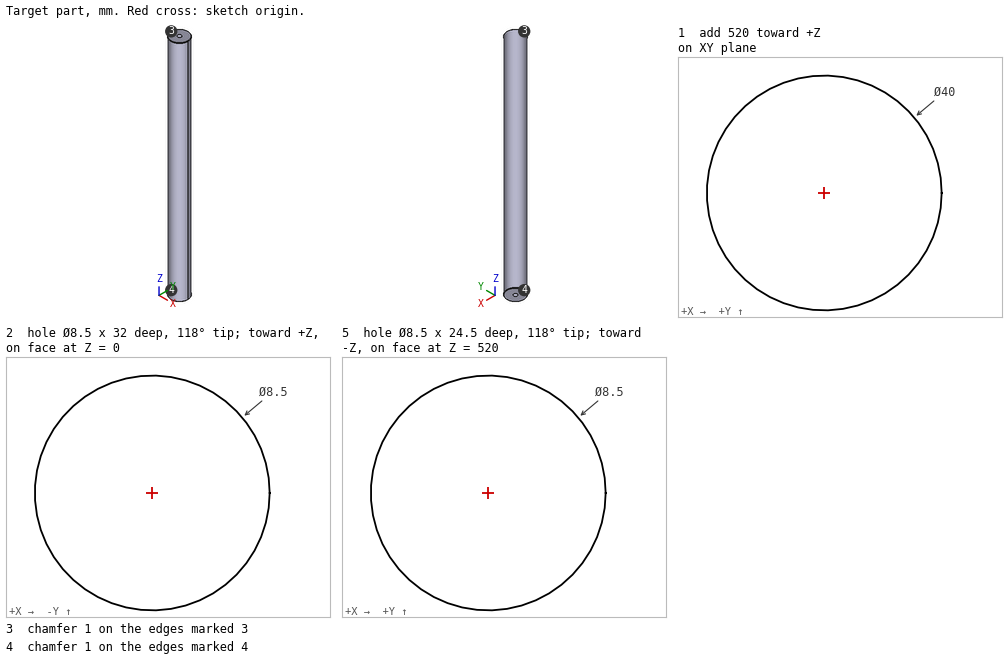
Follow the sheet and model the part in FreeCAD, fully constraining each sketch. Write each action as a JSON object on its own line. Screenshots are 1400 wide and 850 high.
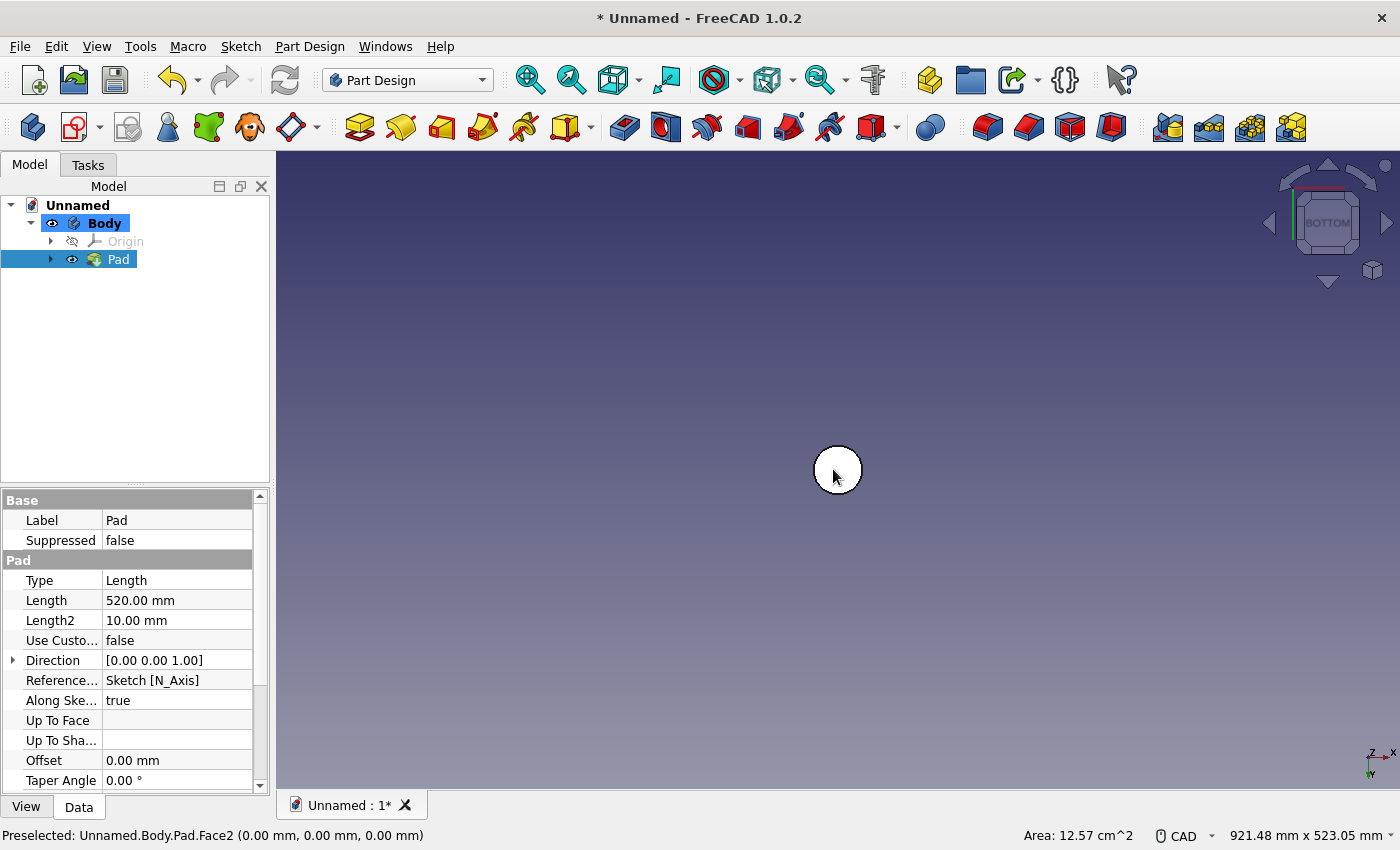
{"action": "left_click", "coordinate": [74, 128]}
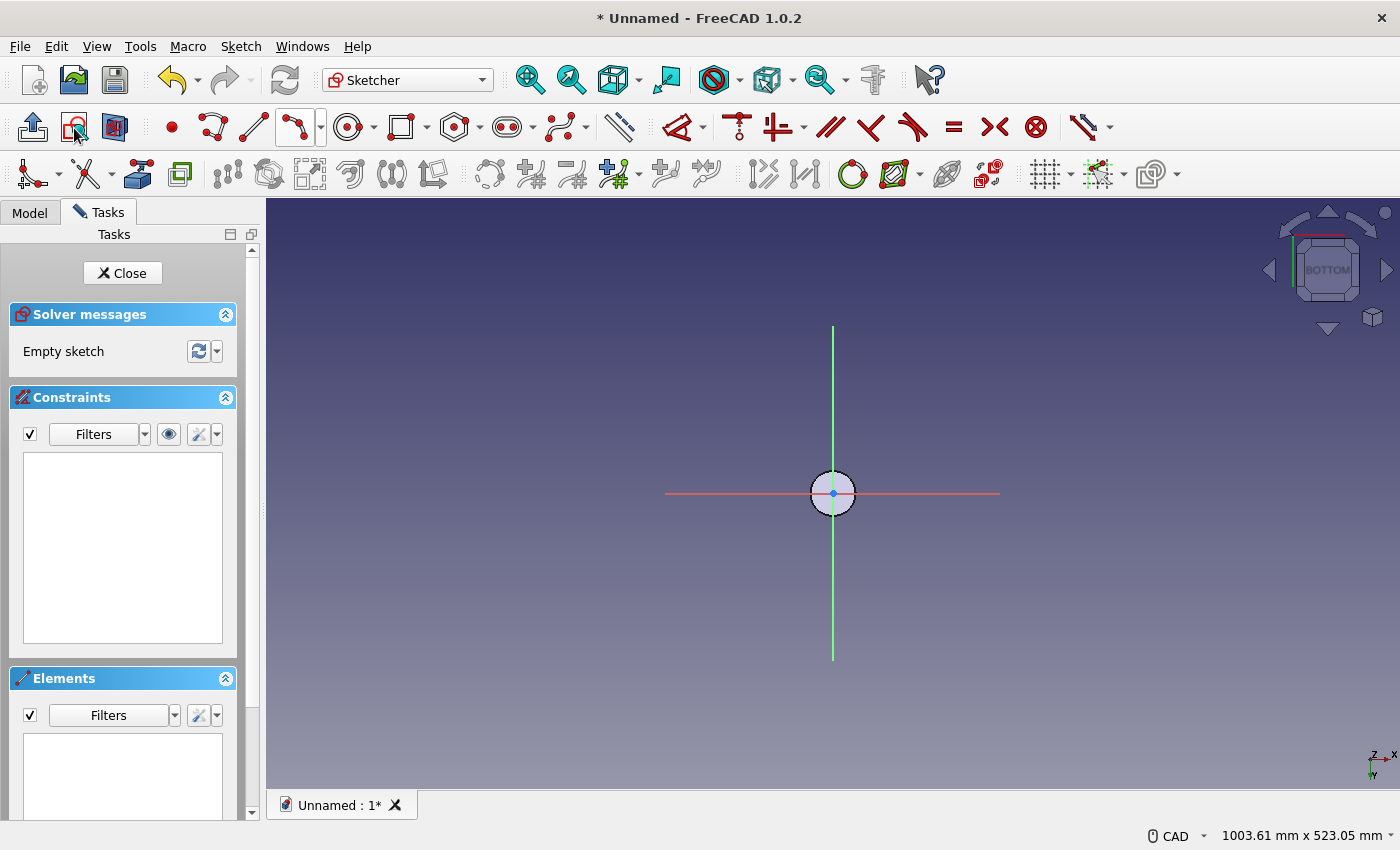
{"action": "scroll", "coordinate": [837, 494], "scroll_direction": "up", "scroll_amount": 15}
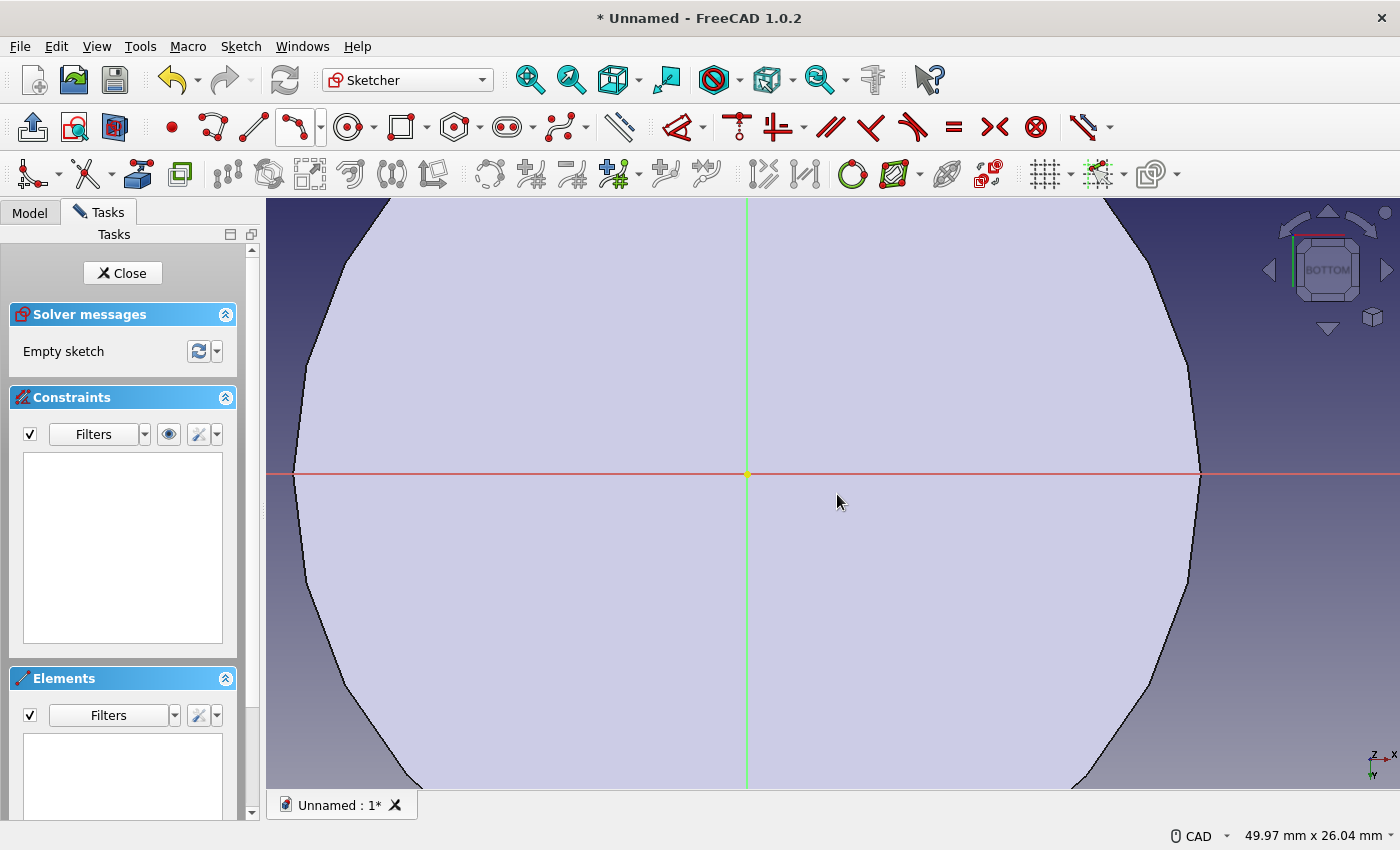
{"action": "scroll", "coordinate": [726, 451], "scroll_direction": "up", "scroll_amount": 3}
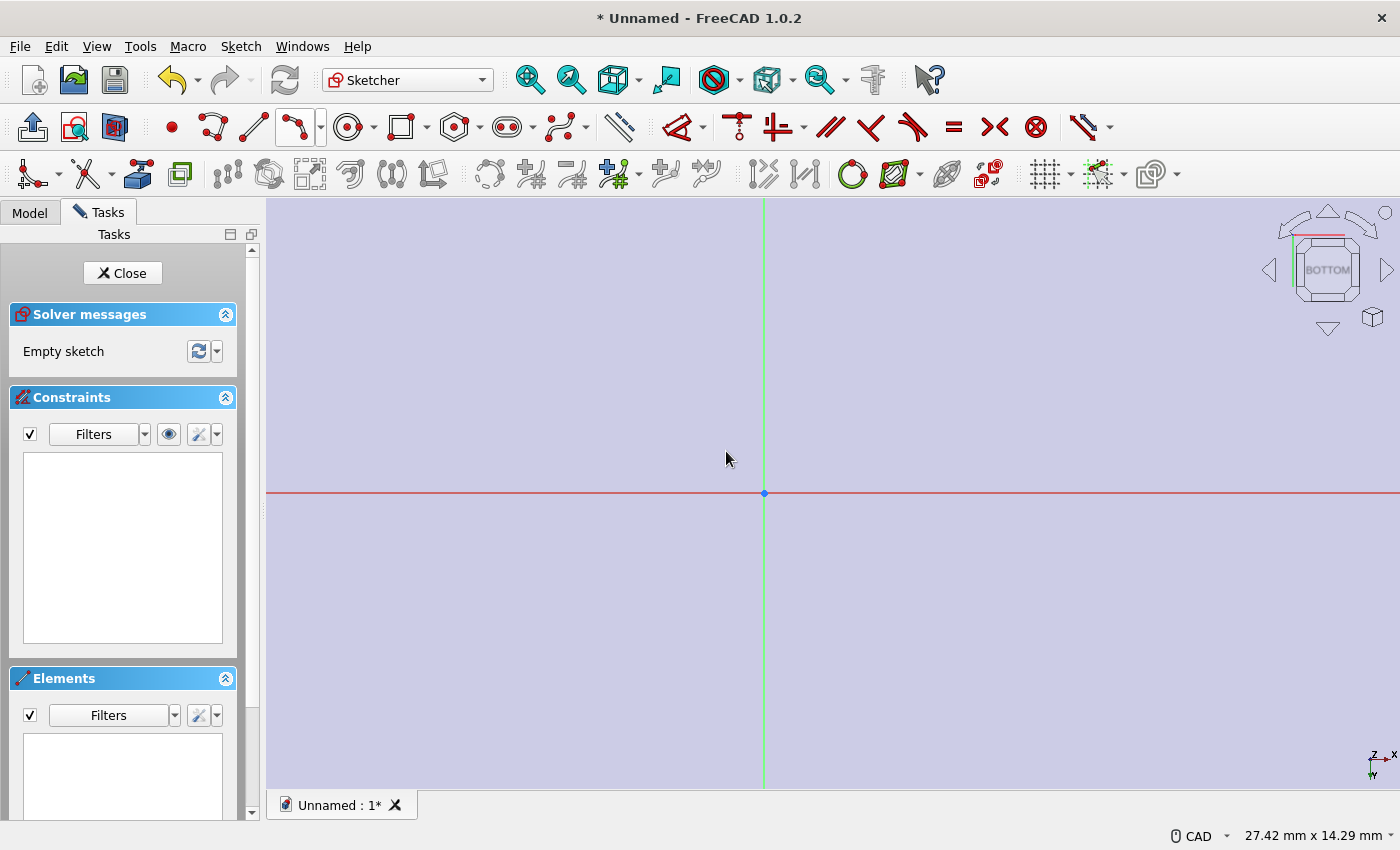
{"action": "left_click", "coordinate": [348, 128]}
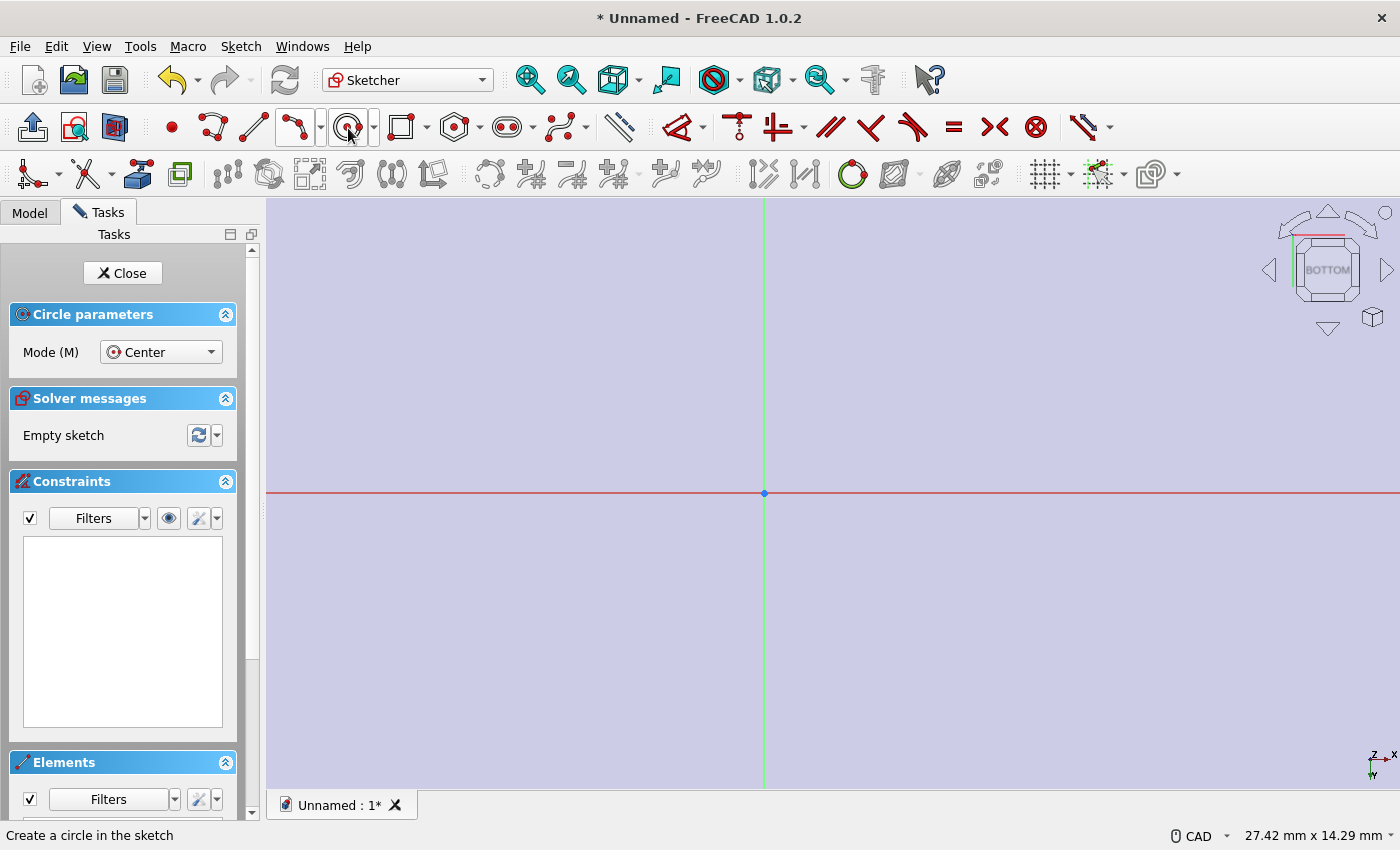
{"action": "left_click", "coordinate": [764, 493]}
{"action": "left_click", "coordinate": [888, 369]}
{"action": "key", "text": "Escape"}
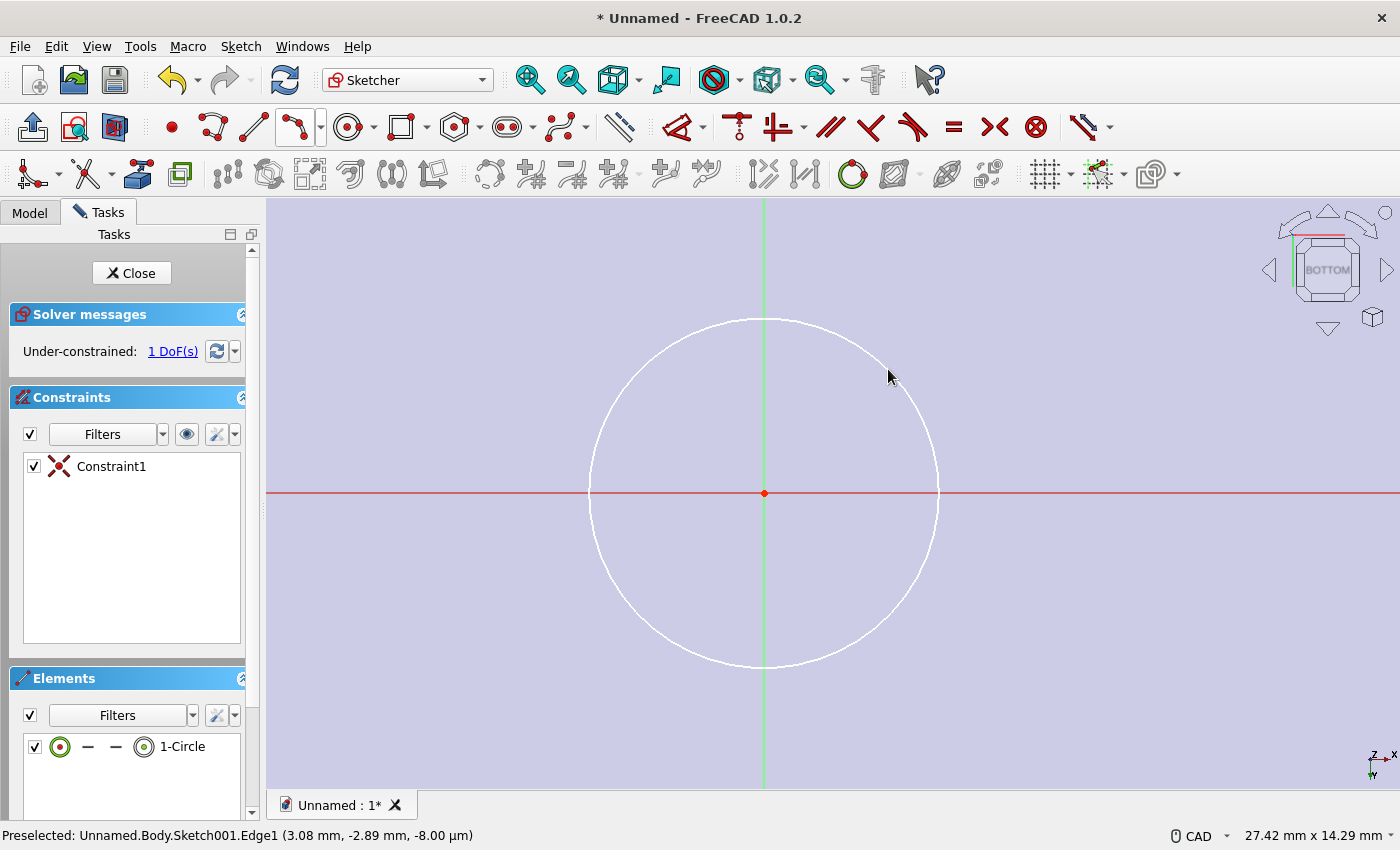
{"action": "left_click", "coordinate": [676, 128]}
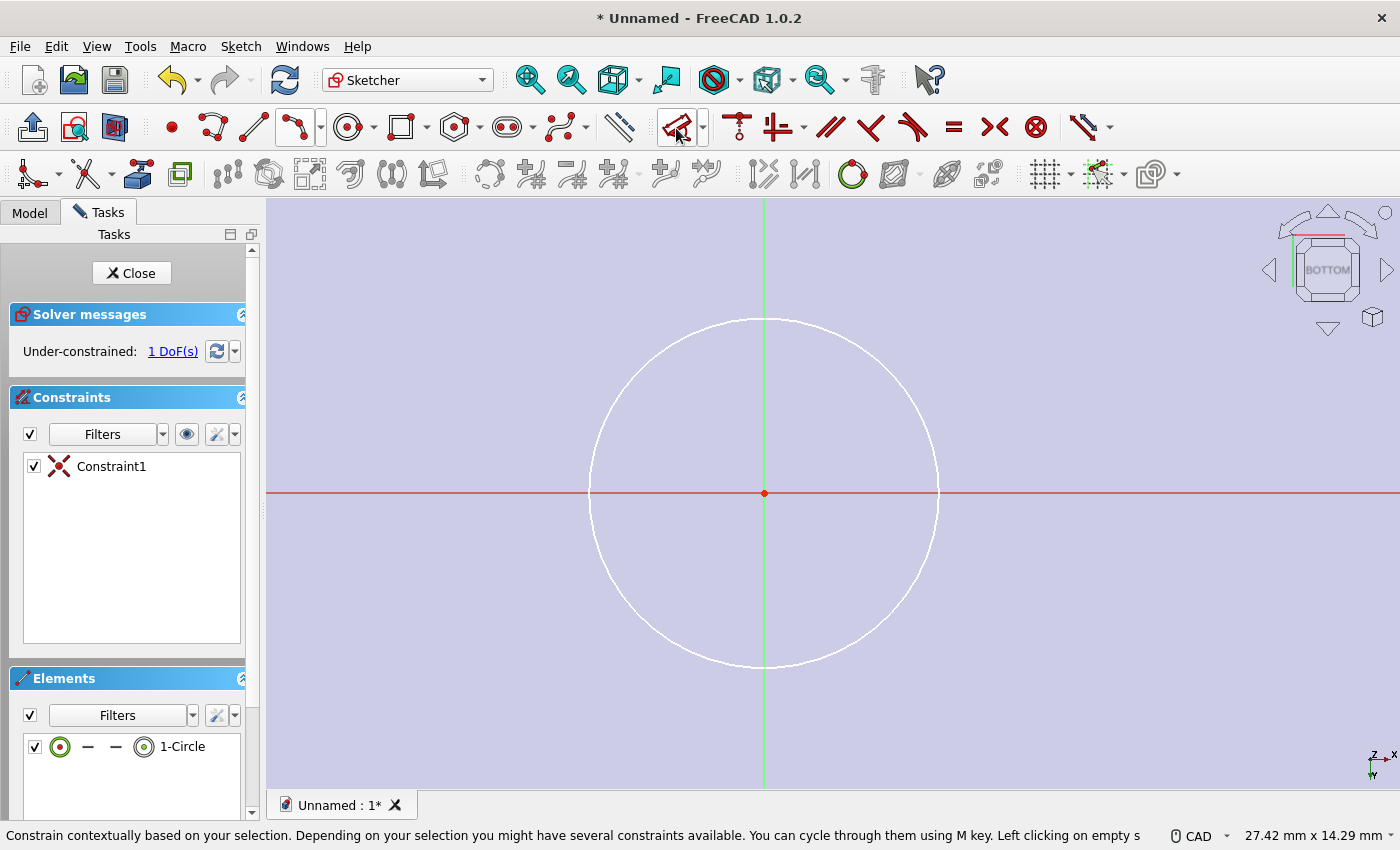
{"action": "left_click", "coordinate": [887, 369]}
{"action": "left_click", "coordinate": [910, 346]}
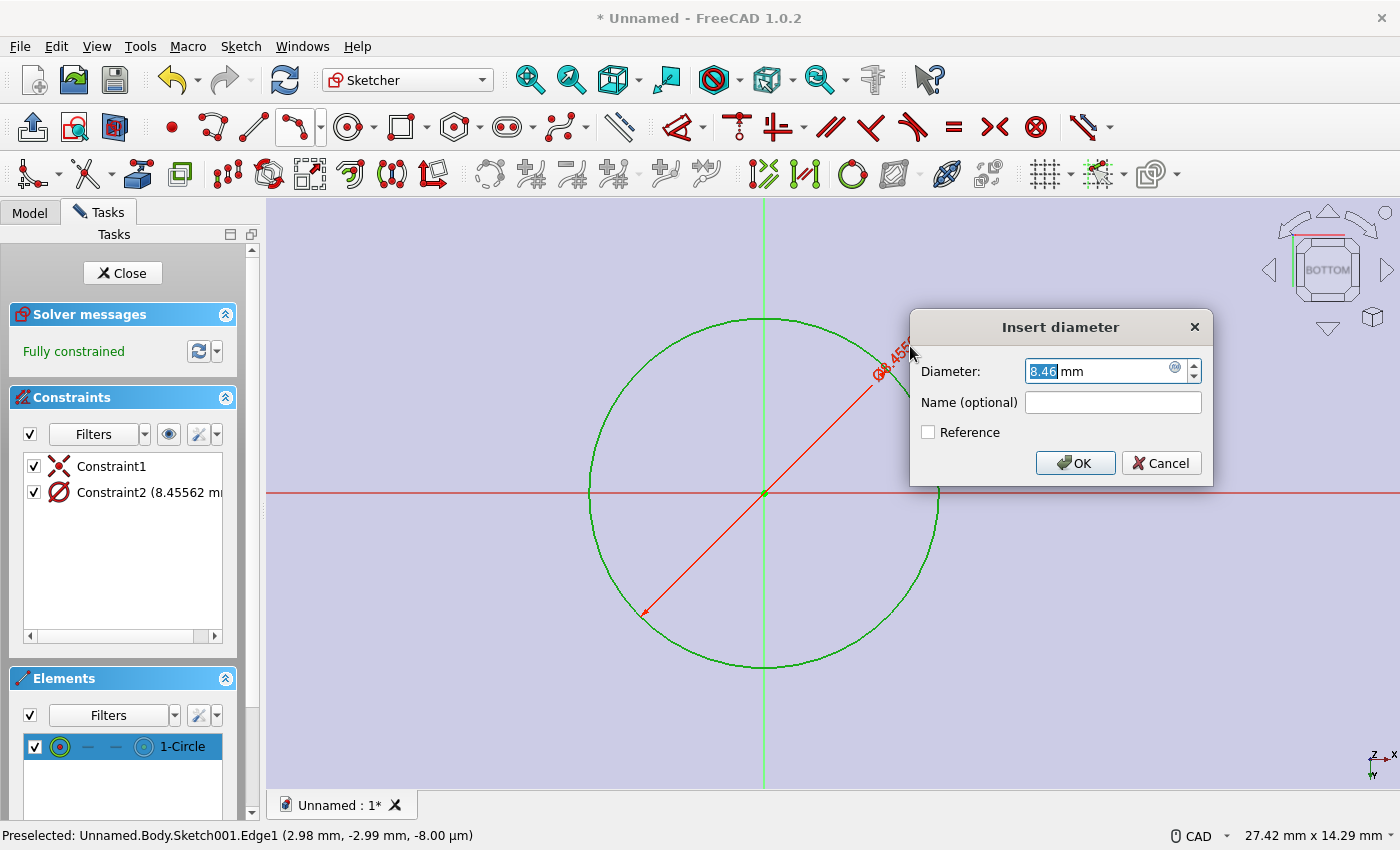
{"action": "type", "text": "8.5"}
{"action": "key", "text": "Return"}
{"action": "key", "text": "Escape"}